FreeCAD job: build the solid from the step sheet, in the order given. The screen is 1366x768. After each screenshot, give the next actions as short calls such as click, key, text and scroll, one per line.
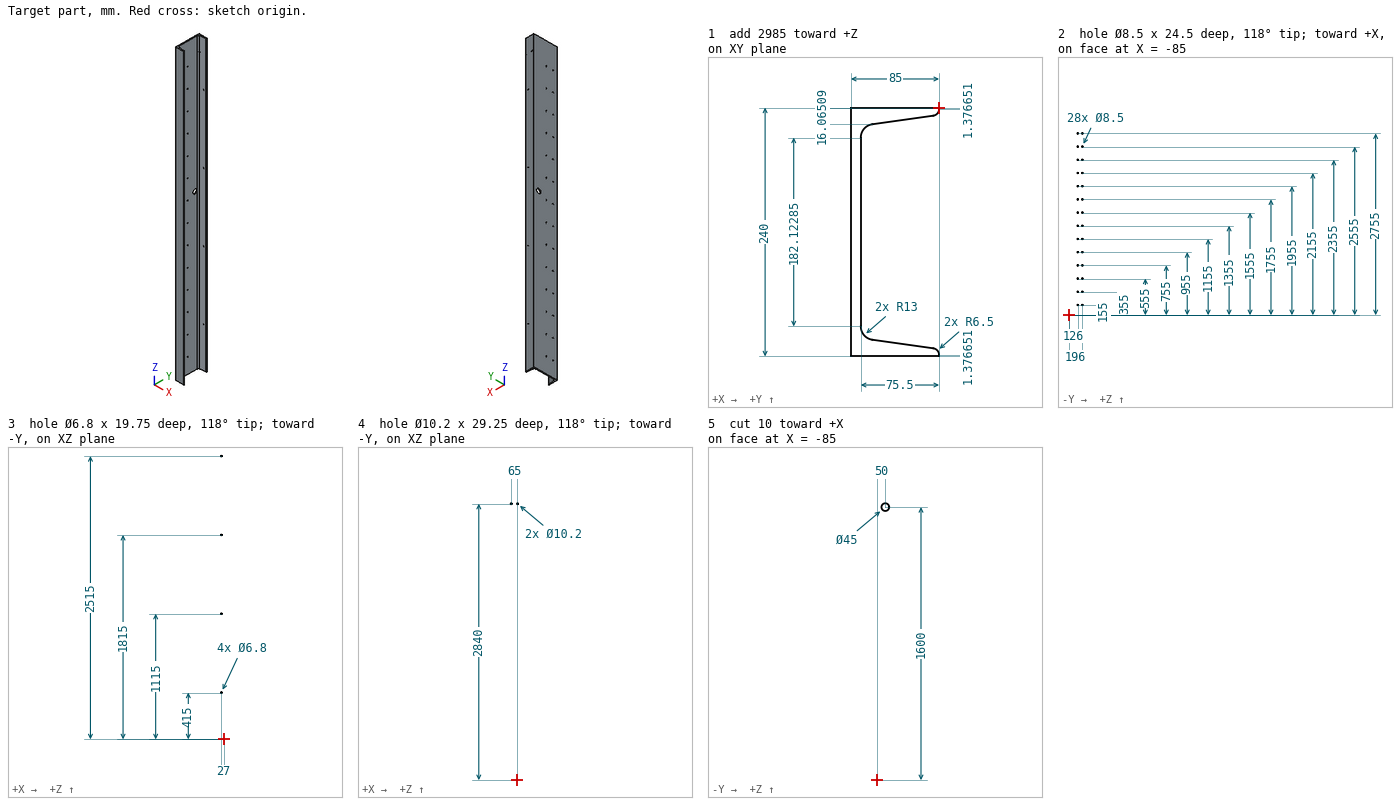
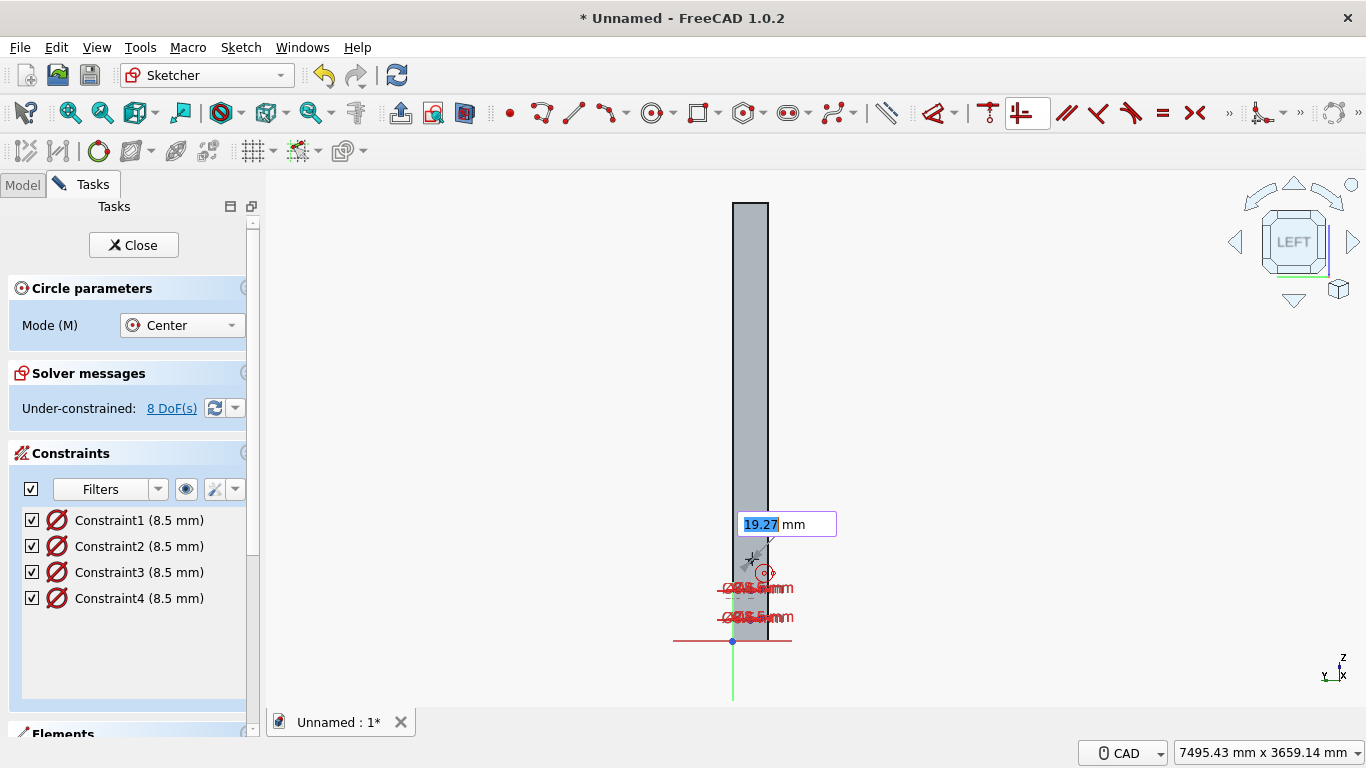
text(8.5)
key(Return)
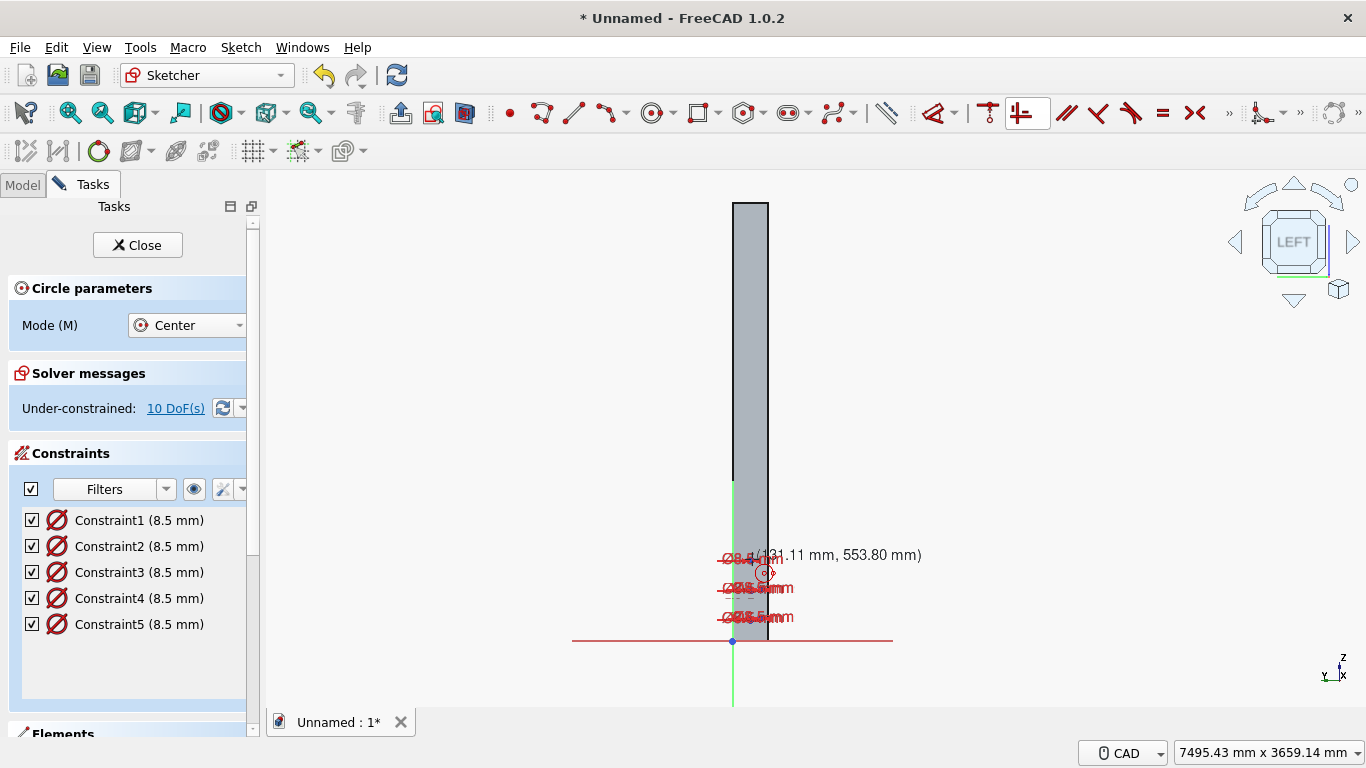
scroll(762, 560, up, 18)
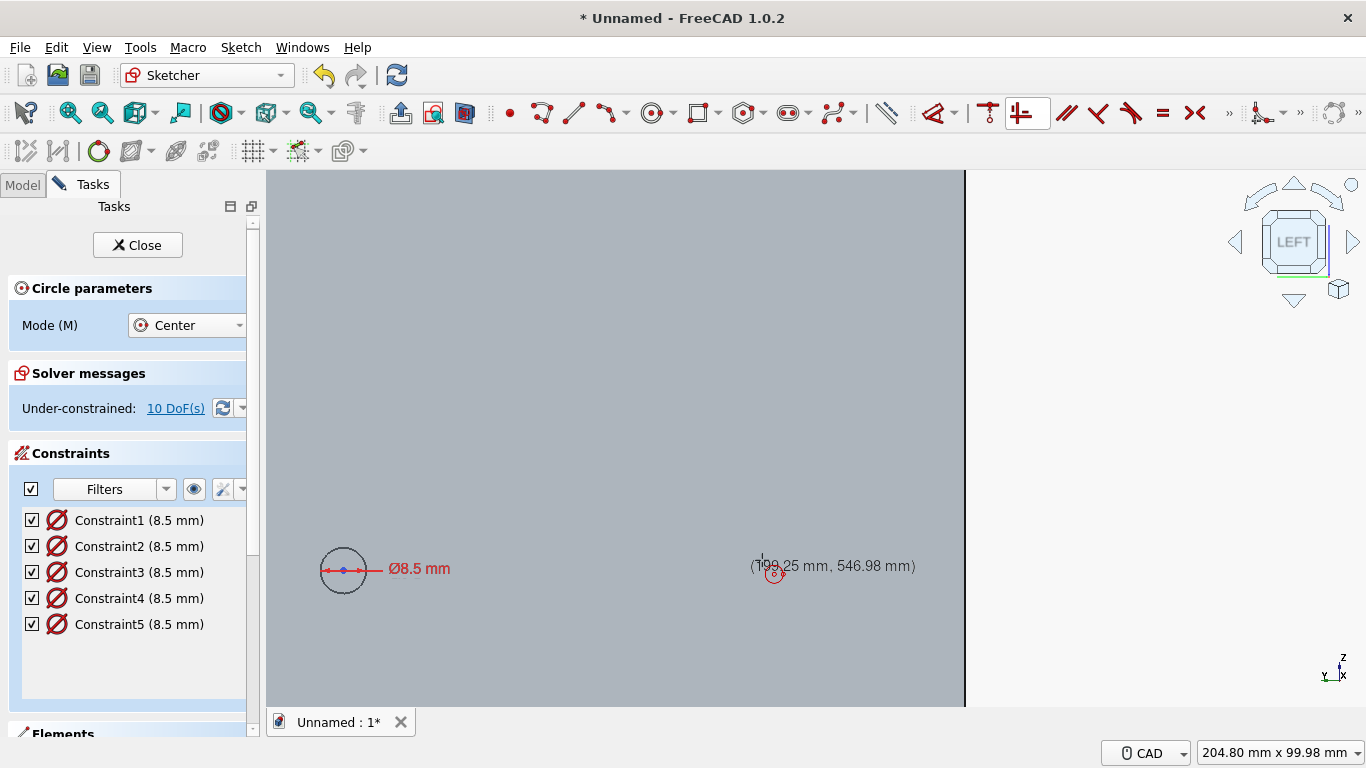
scroll(762, 560, down, 18)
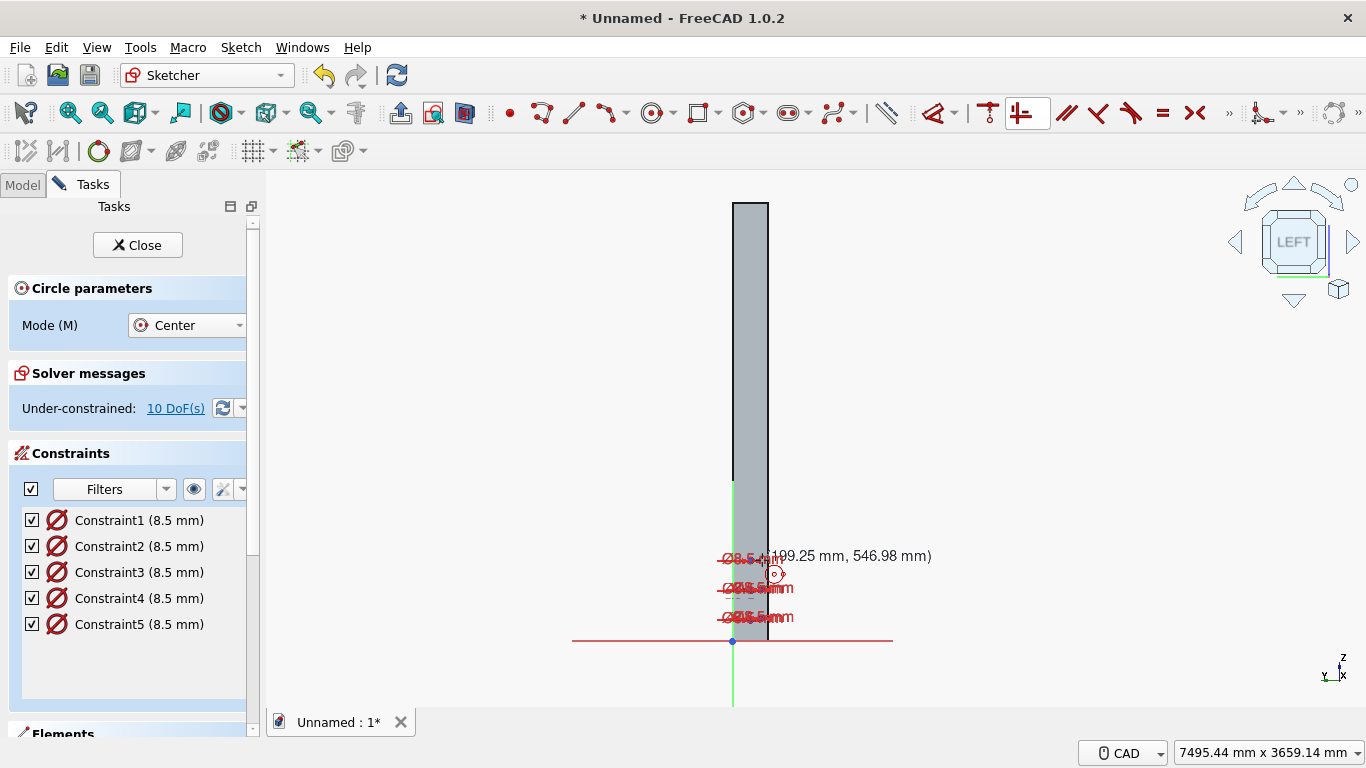
scroll(762, 560, up, 3)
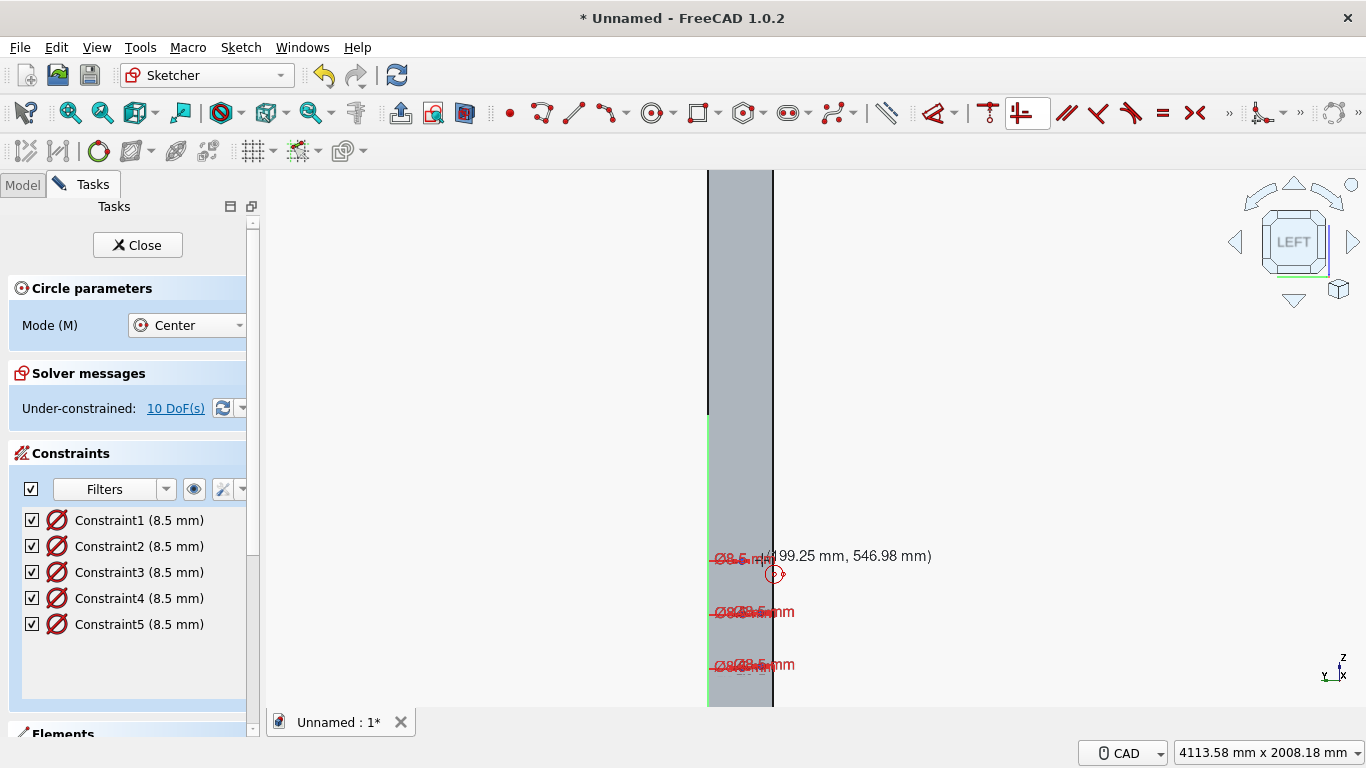
click(761, 559)
move(762, 558)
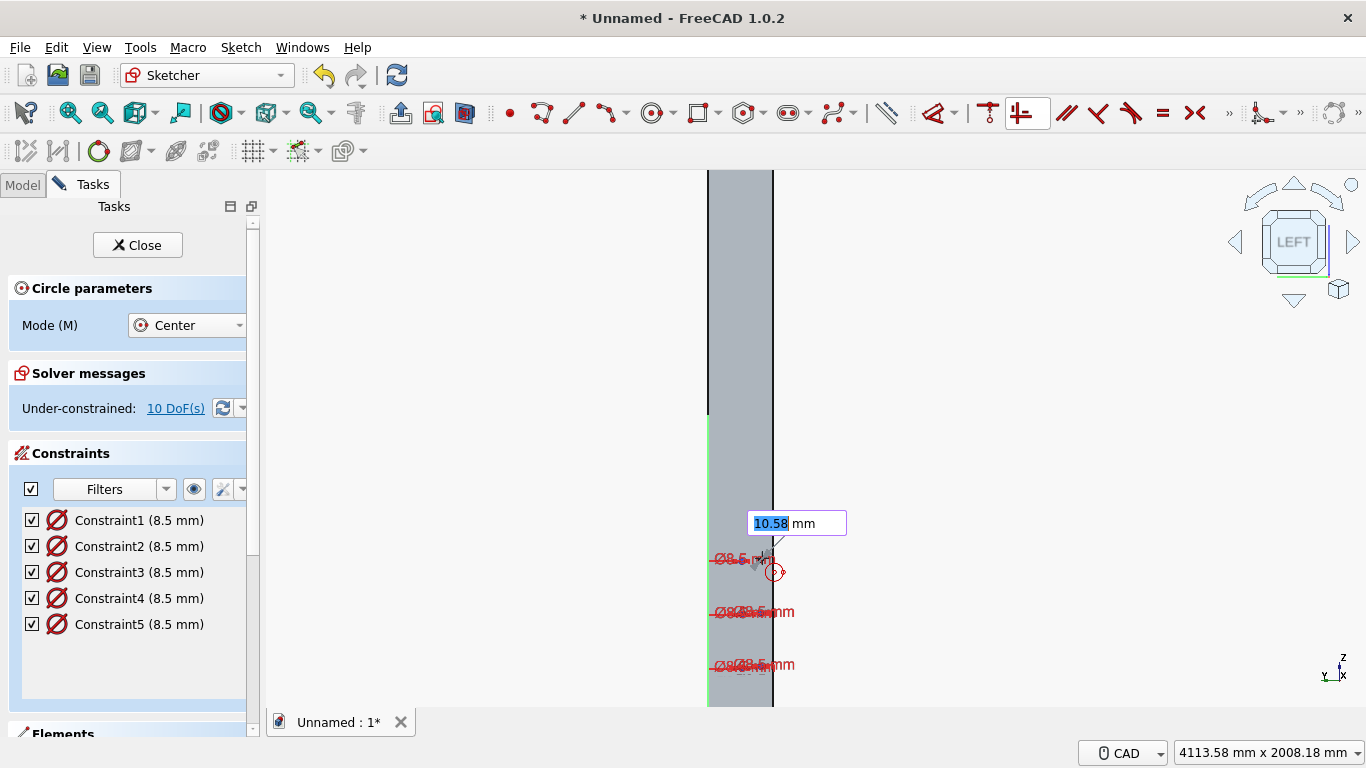
text(8.5)
key(Return)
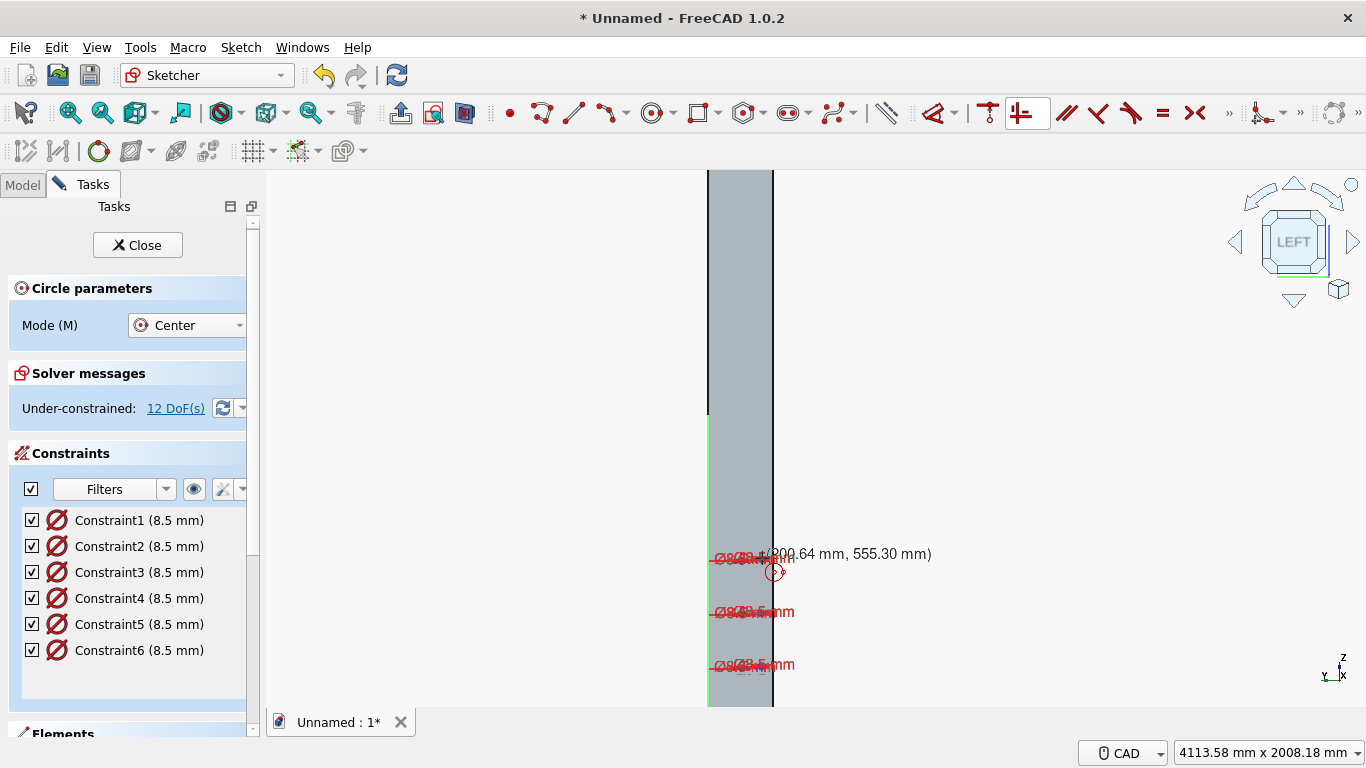
scroll(742, 506, up, 15)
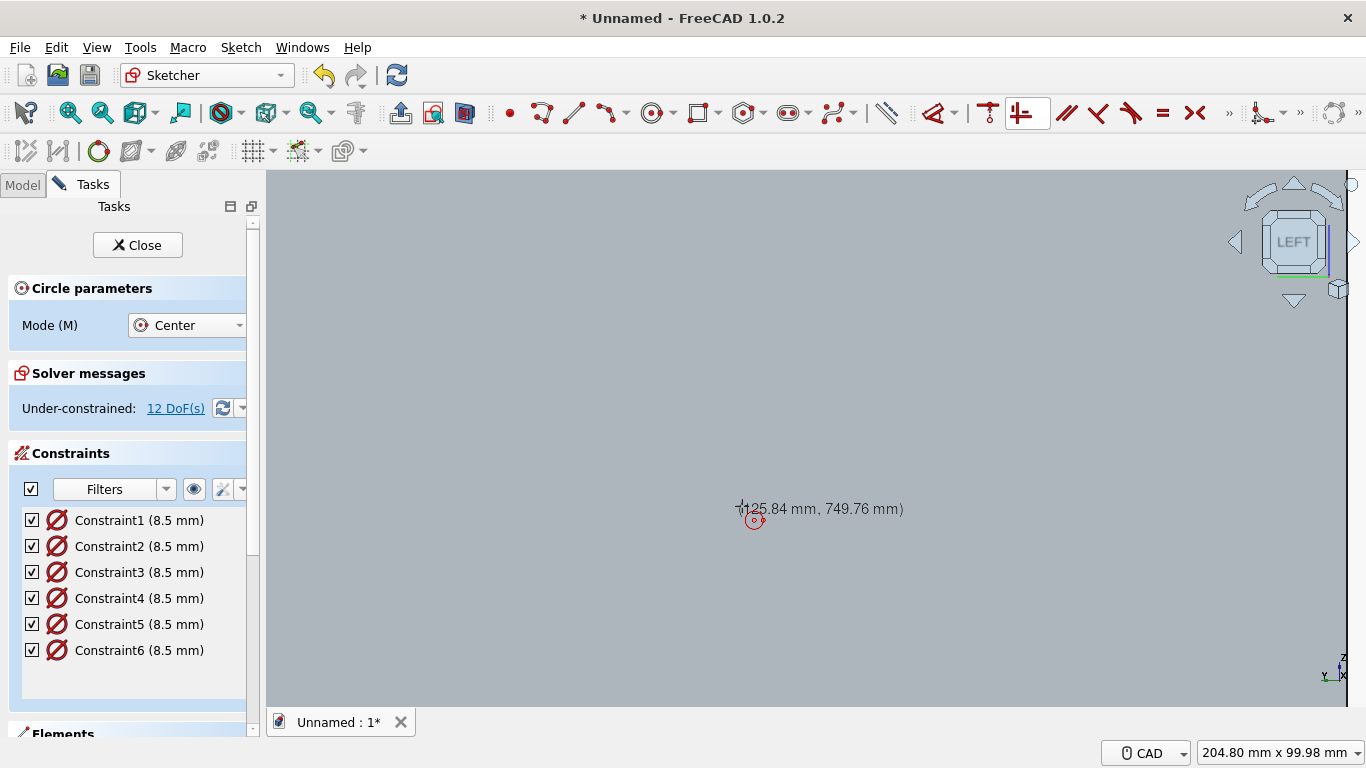
scroll(752, 531, down, 18)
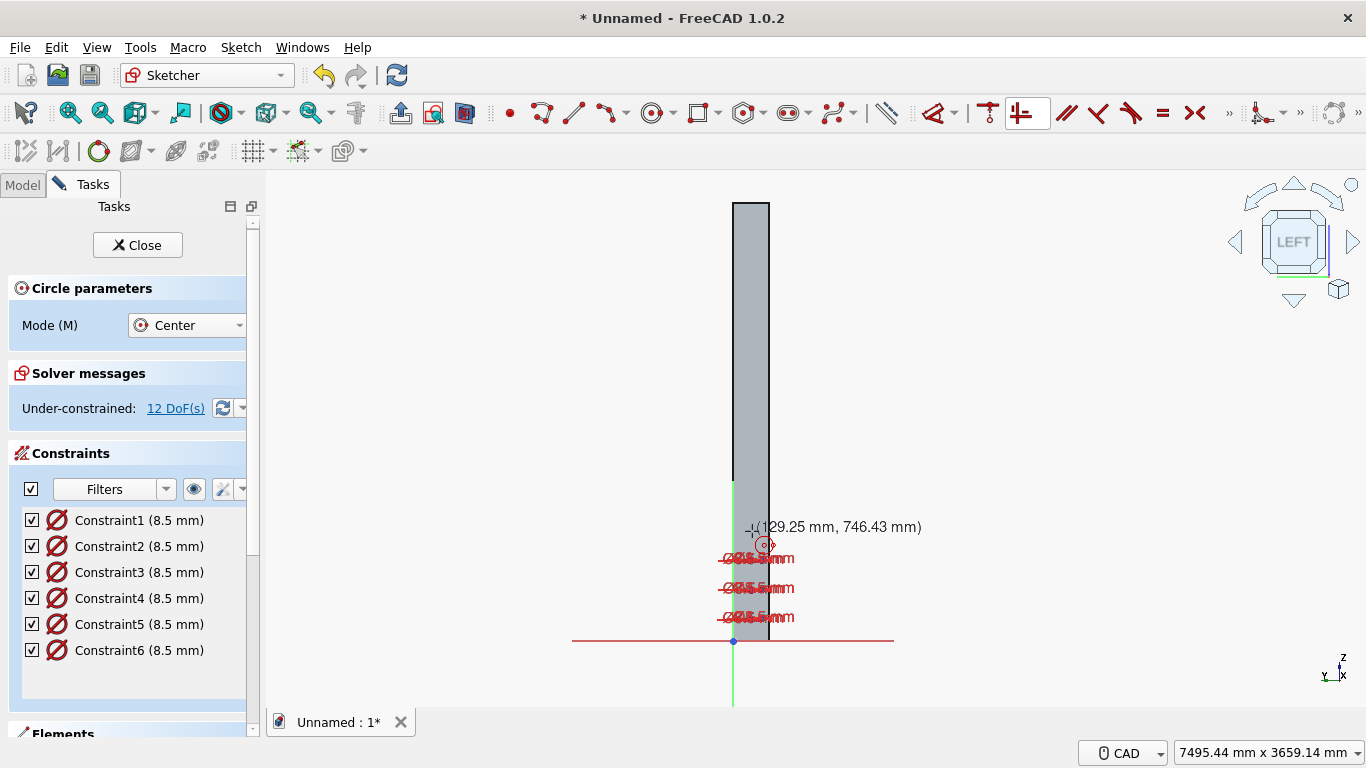
click(752, 530)
move(752, 530)